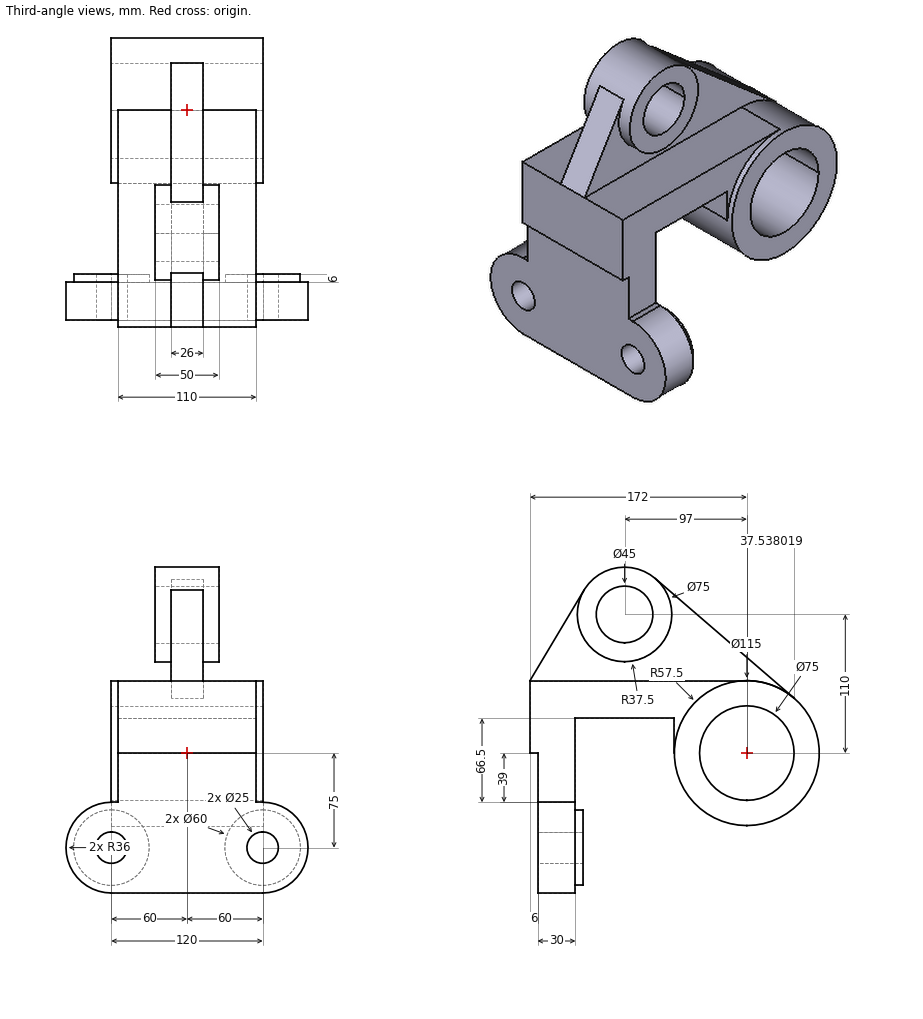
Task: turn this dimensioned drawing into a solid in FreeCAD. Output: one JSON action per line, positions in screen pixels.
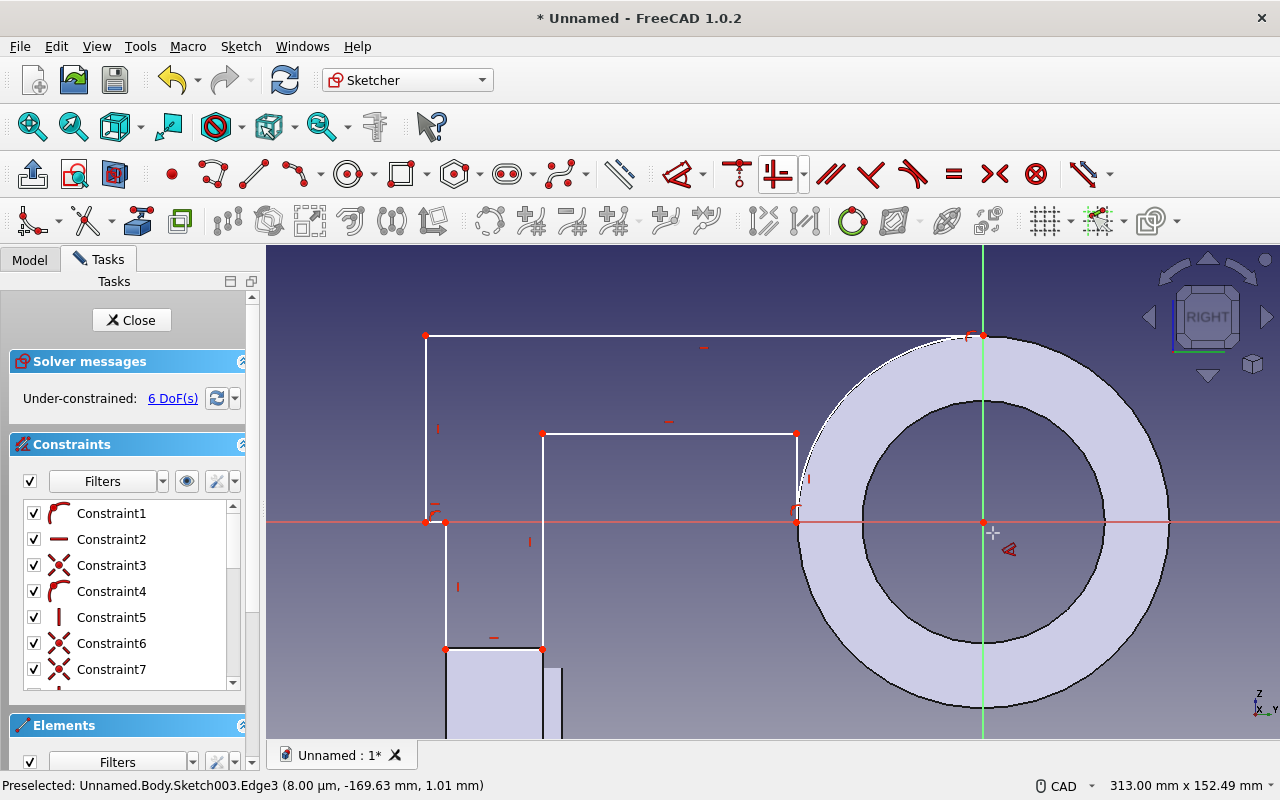
{"action": "left_click", "coordinate": [899, 356]}
{"action": "left_click", "coordinate": [803, 399]}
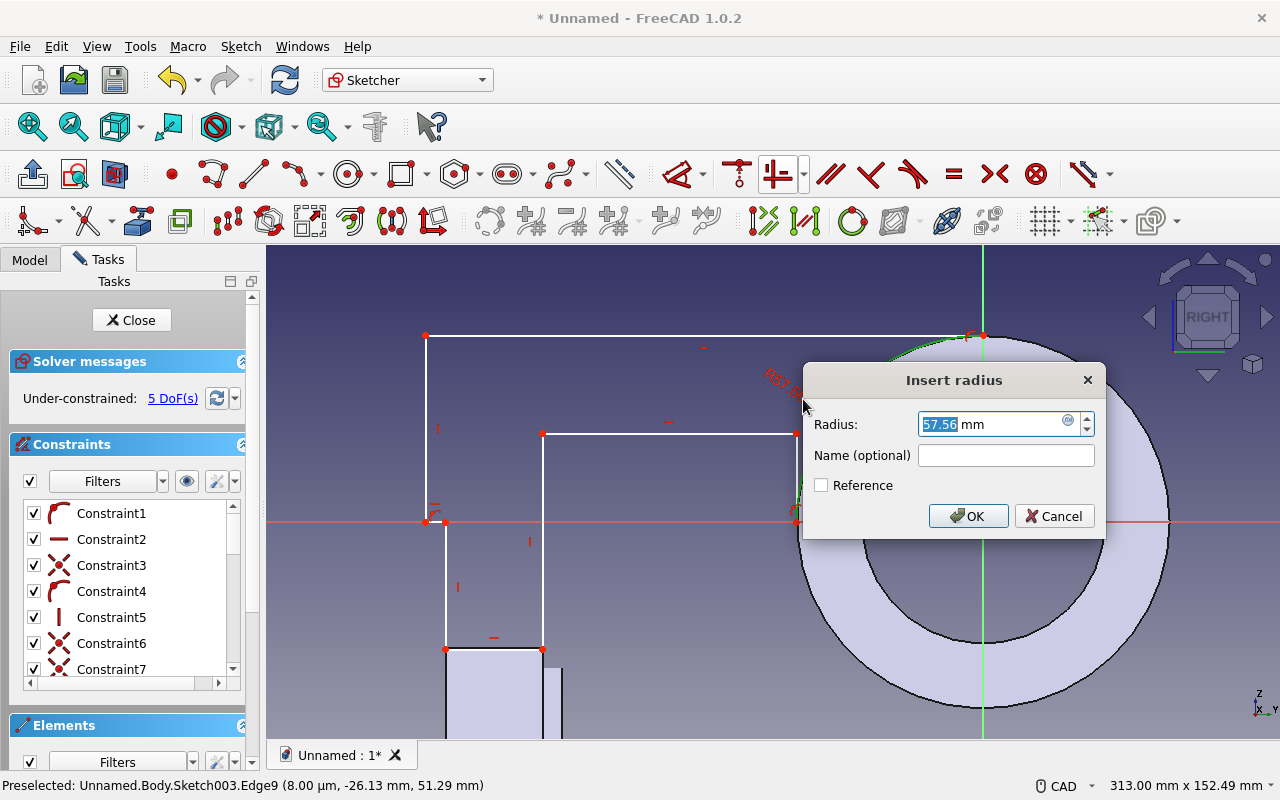
{"action": "type", "text": "57.5"}
{"action": "key", "text": "Return"}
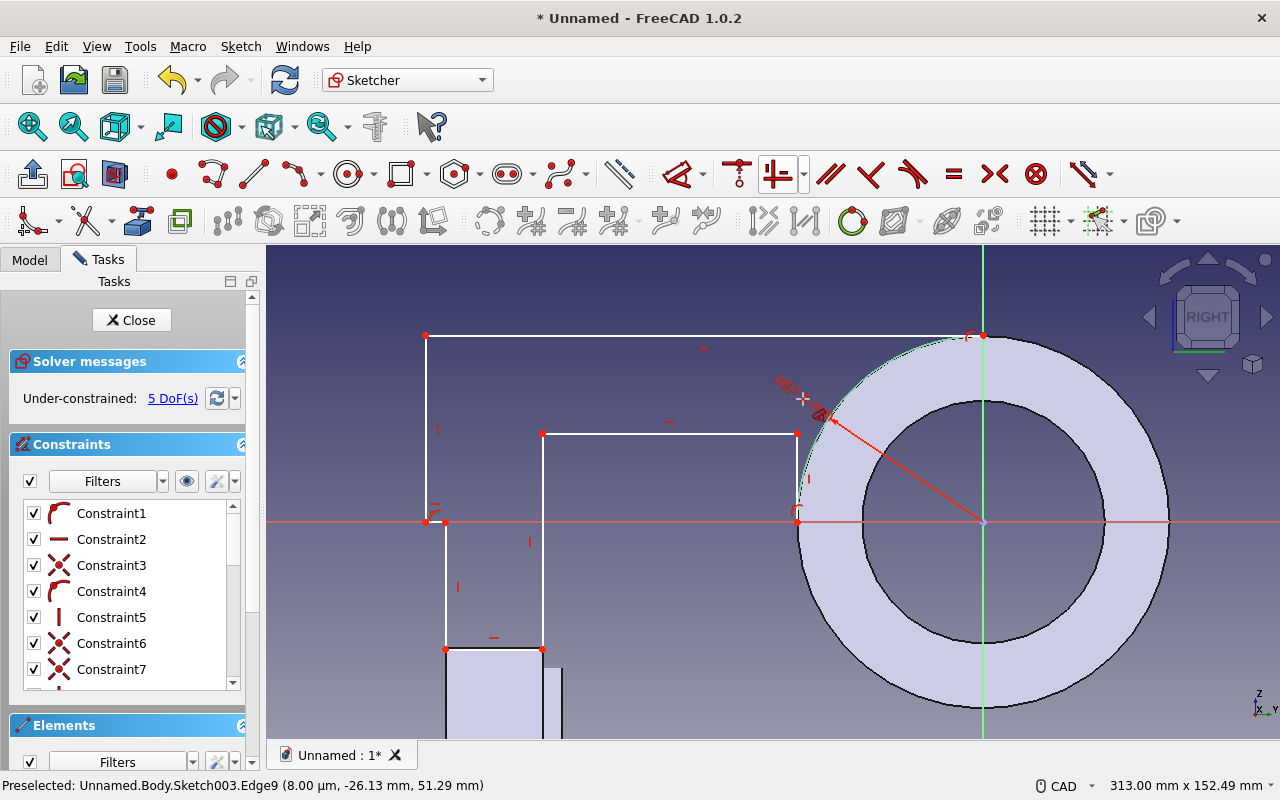
{"action": "scroll", "coordinate": [436, 522], "scroll_direction": "up", "scroll_amount": 4}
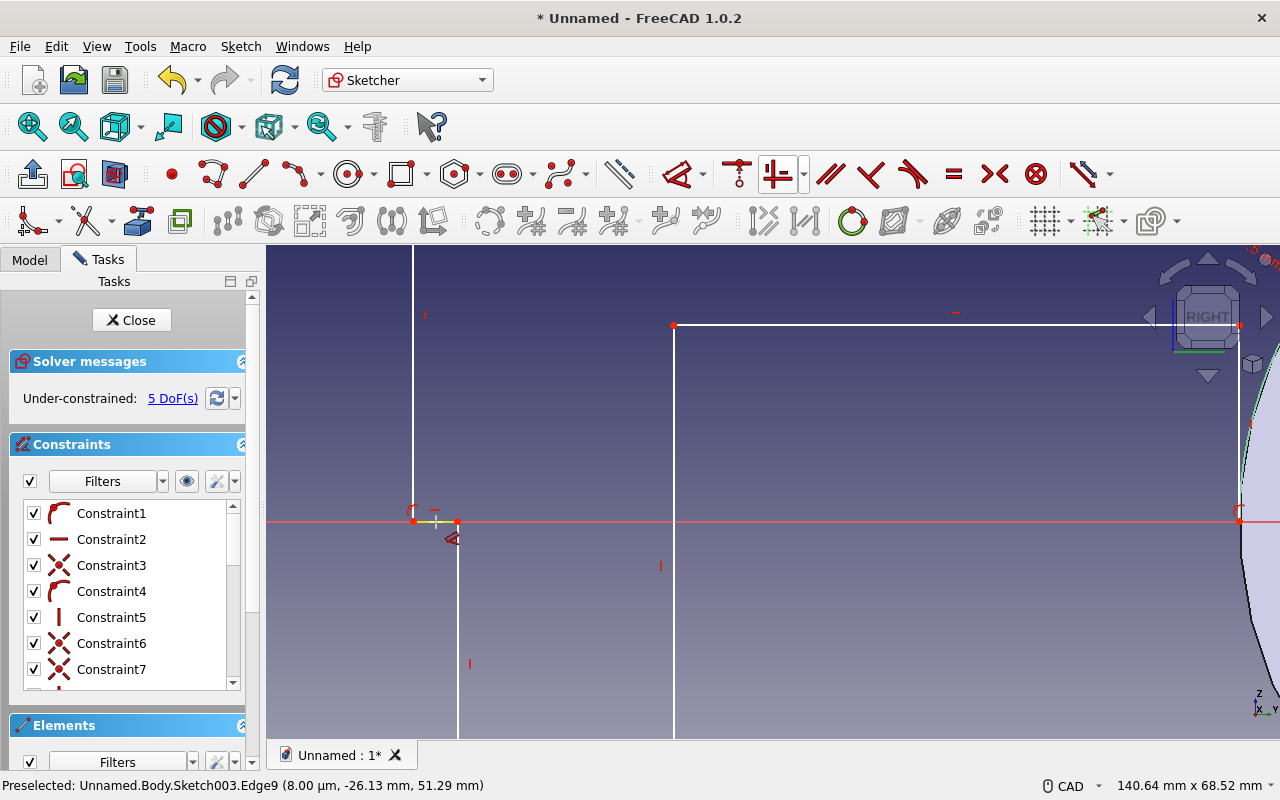
{"action": "left_click", "coordinate": [436, 522]}
{"action": "left_click", "coordinate": [436, 556]}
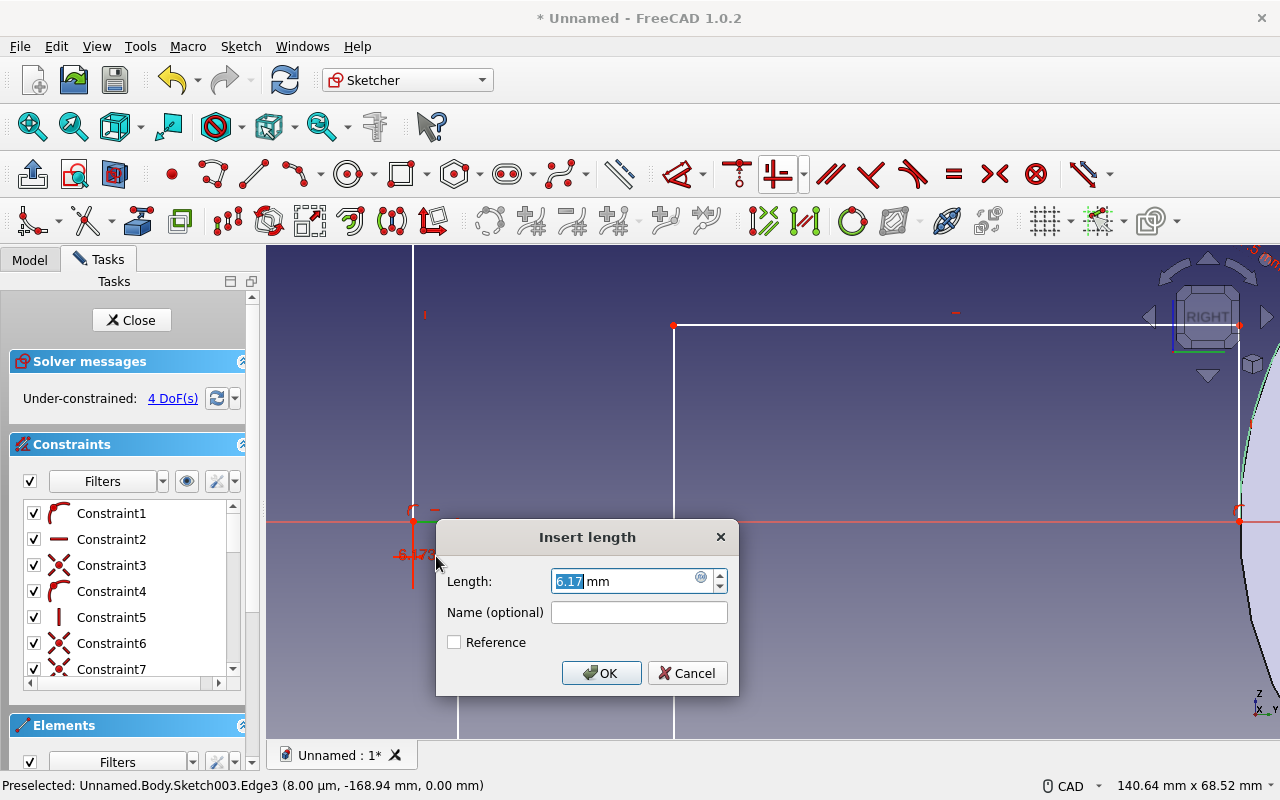
{"action": "type", "text": "6"}
{"action": "key", "text": "Return"}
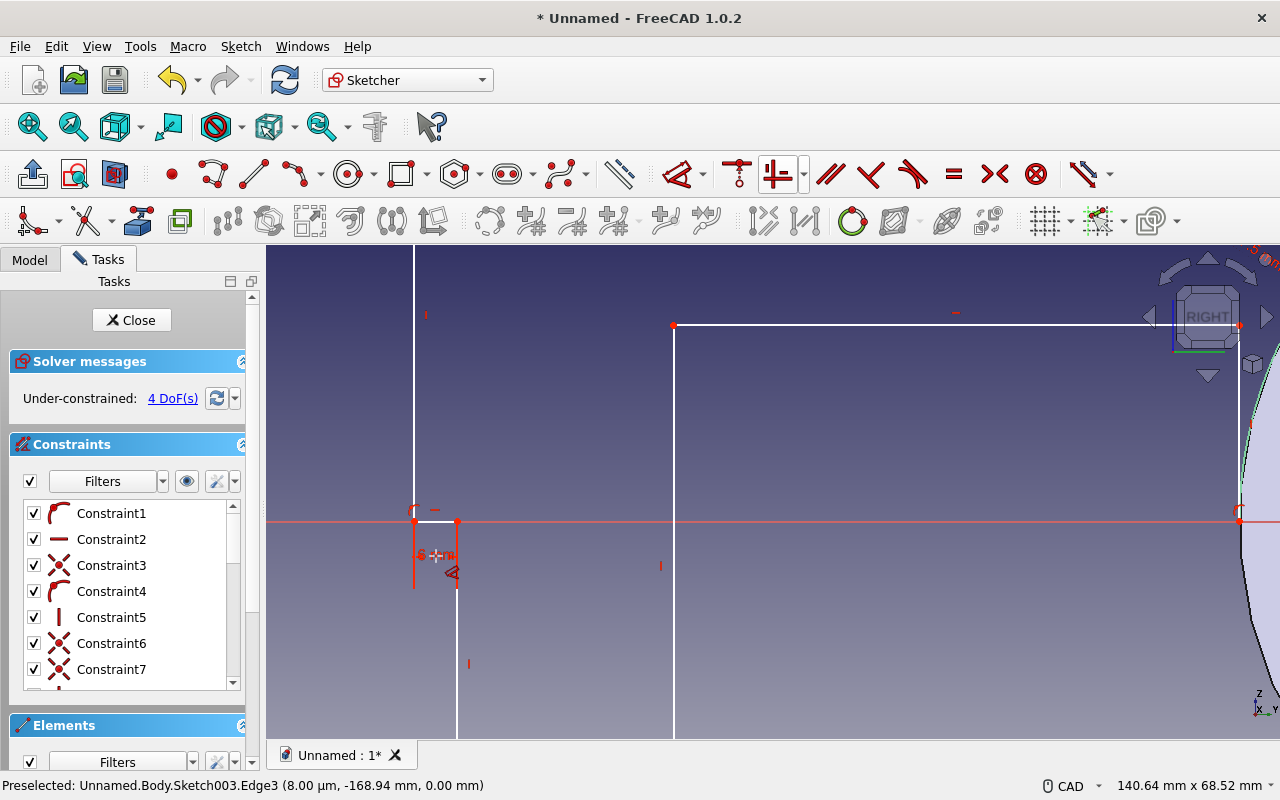
{"action": "left_click", "coordinate": [457, 607]}
{"action": "left_click", "coordinate": [423, 616]}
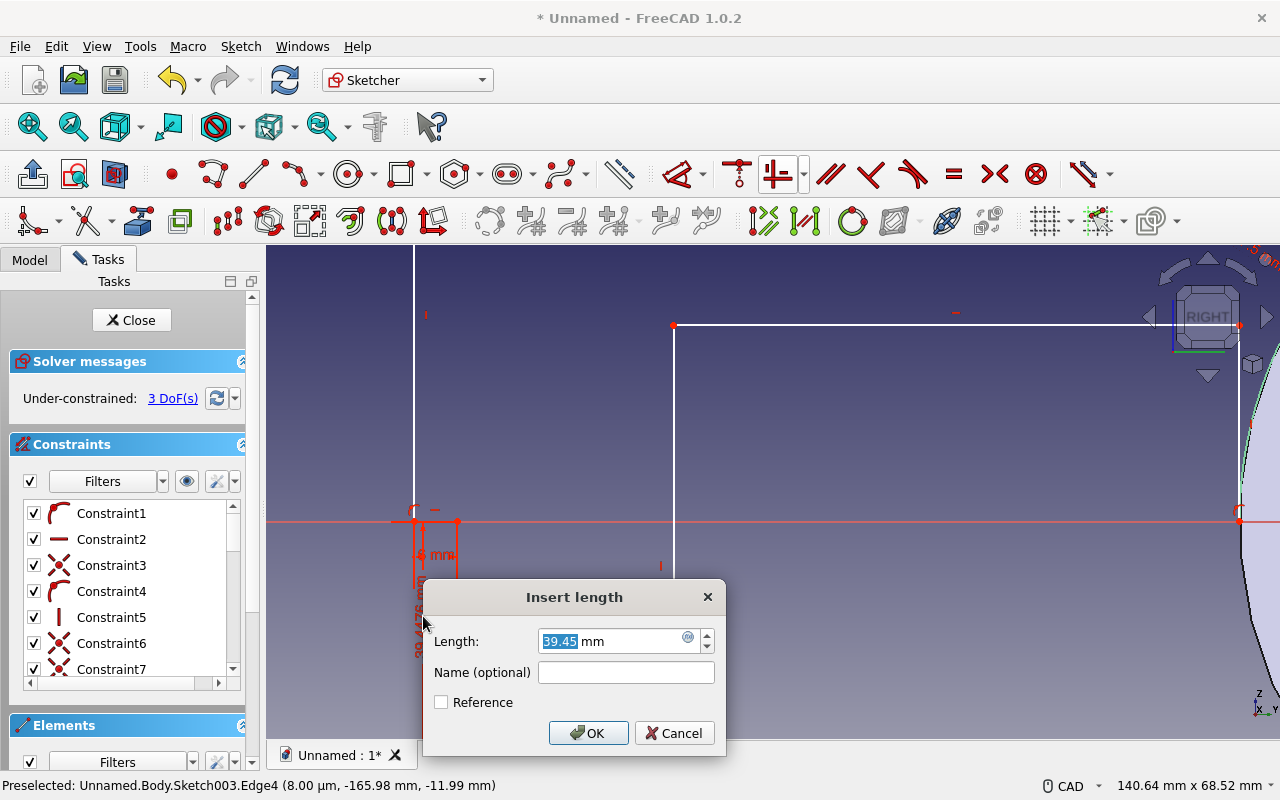
{"action": "type", "text": "39"}
{"action": "key", "text": "Return"}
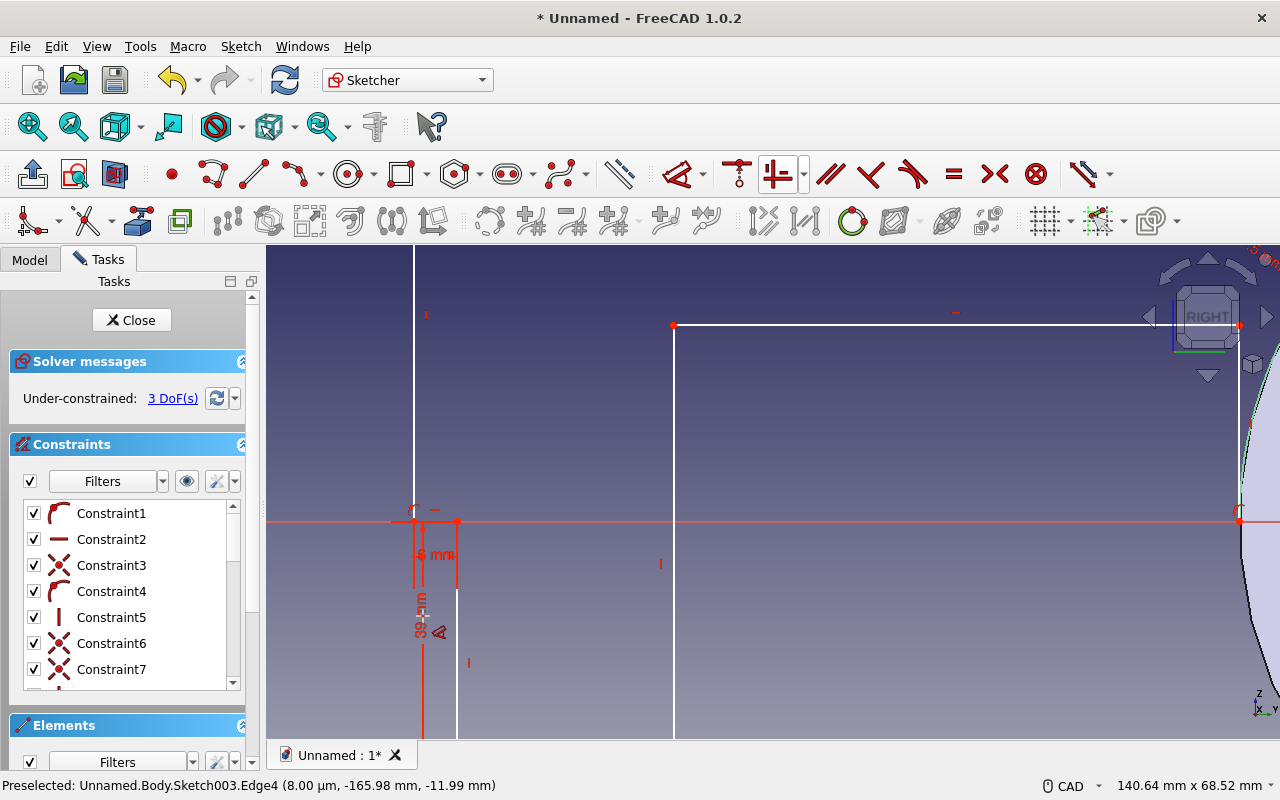
{"action": "scroll", "coordinate": [436, 522], "scroll_direction": "down", "scroll_amount": 4}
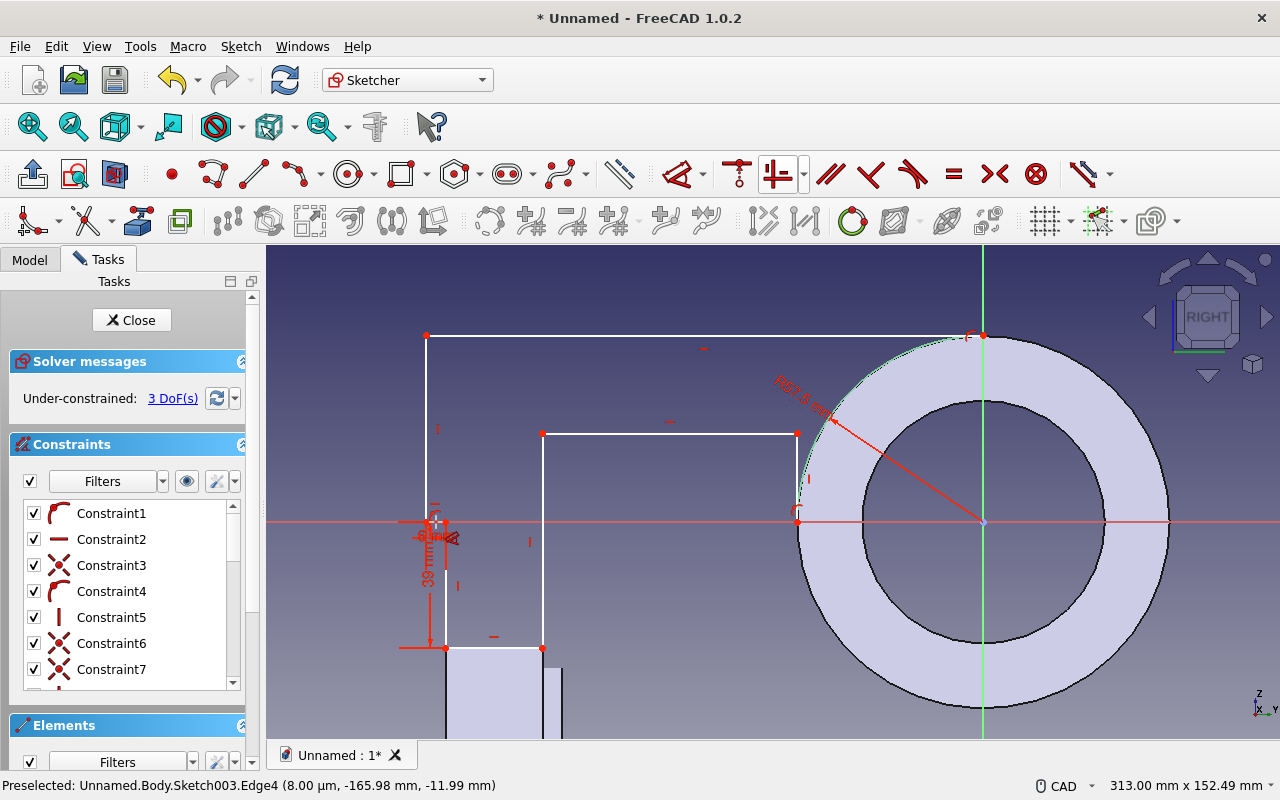
{"action": "left_click", "coordinate": [475, 648]}
{"action": "left_click", "coordinate": [494, 682]}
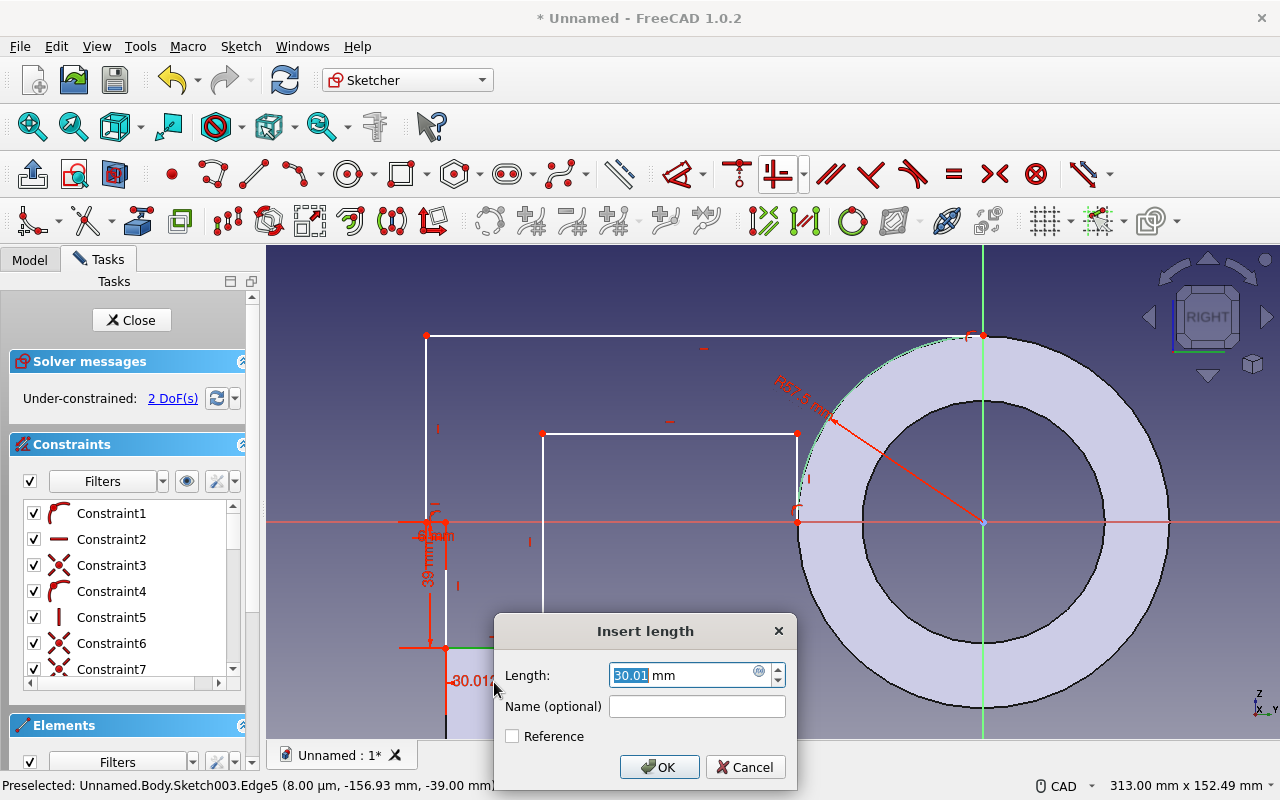
{"action": "type", "text": "30"}
{"action": "key", "text": "Return"}